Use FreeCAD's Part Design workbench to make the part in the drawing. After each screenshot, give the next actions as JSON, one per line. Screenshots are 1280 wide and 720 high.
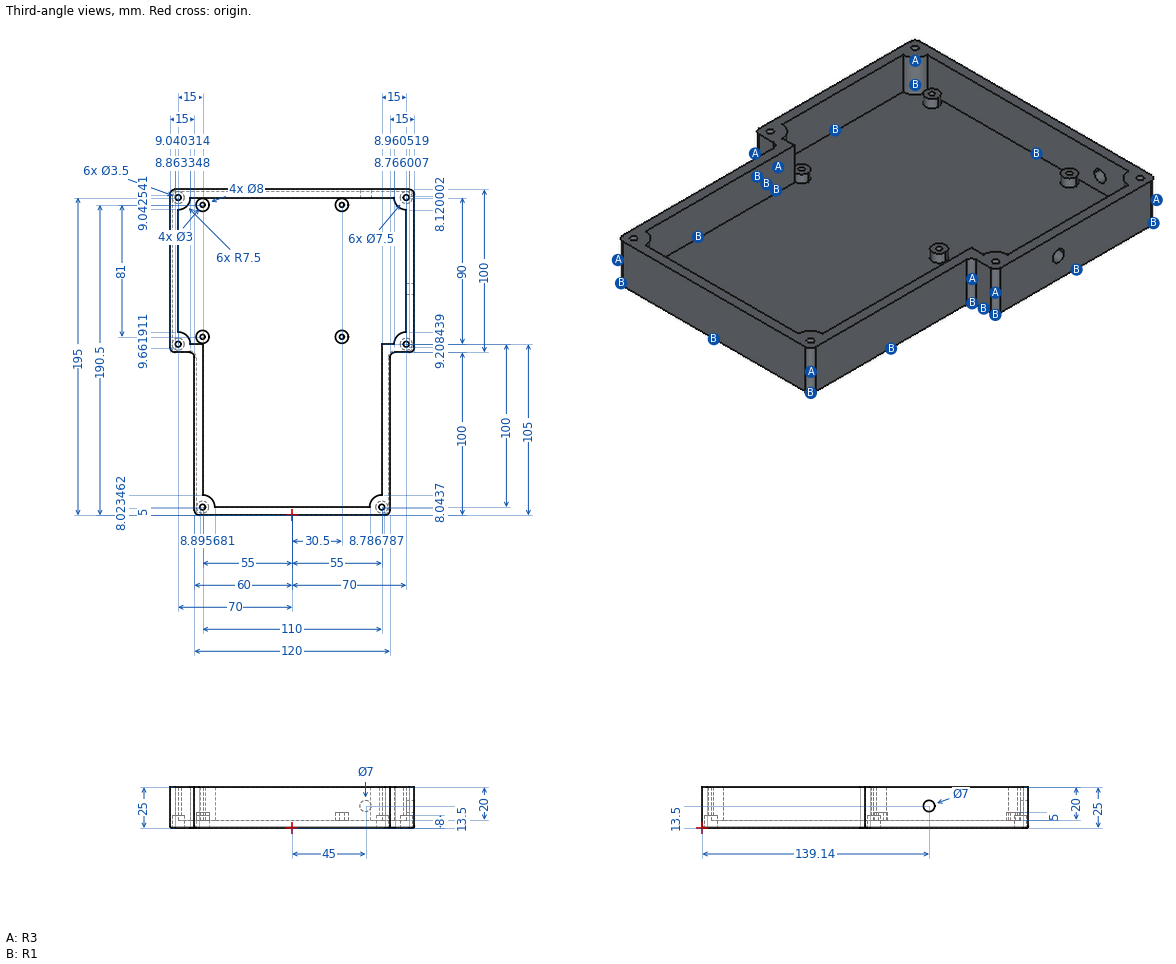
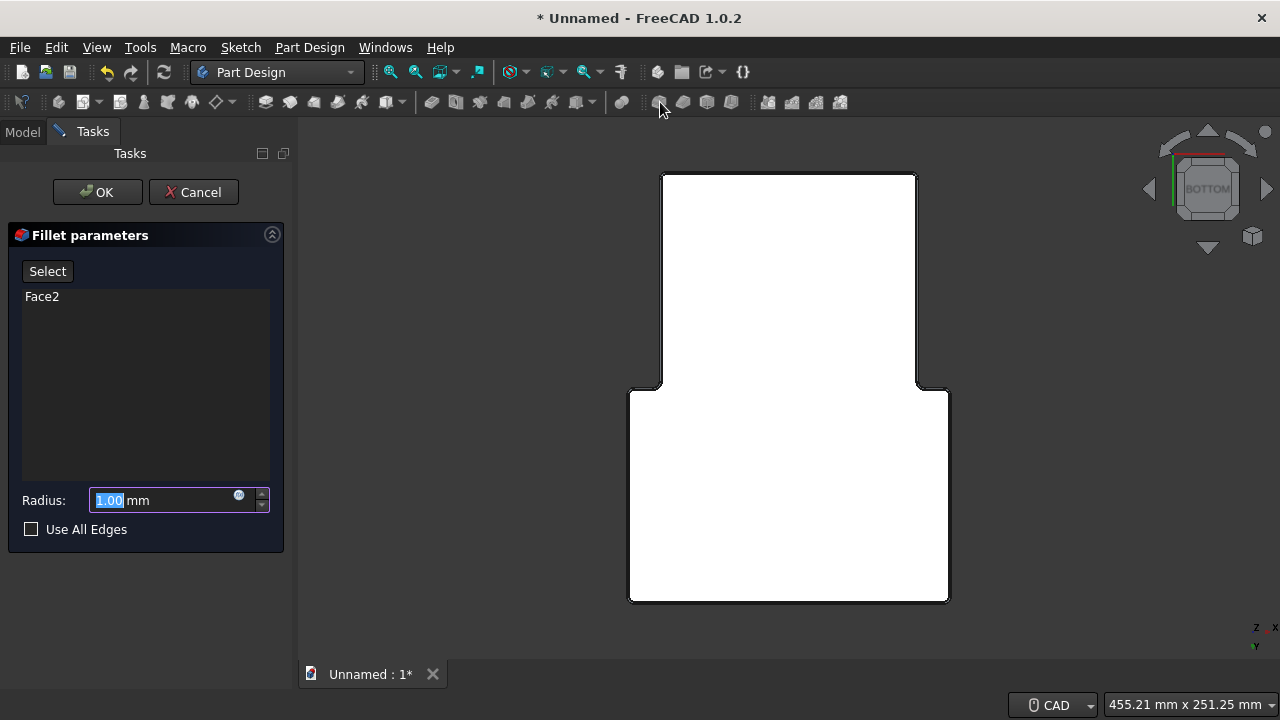
{"action": "type", "text": "1"}
{"action": "key", "text": "Tab"}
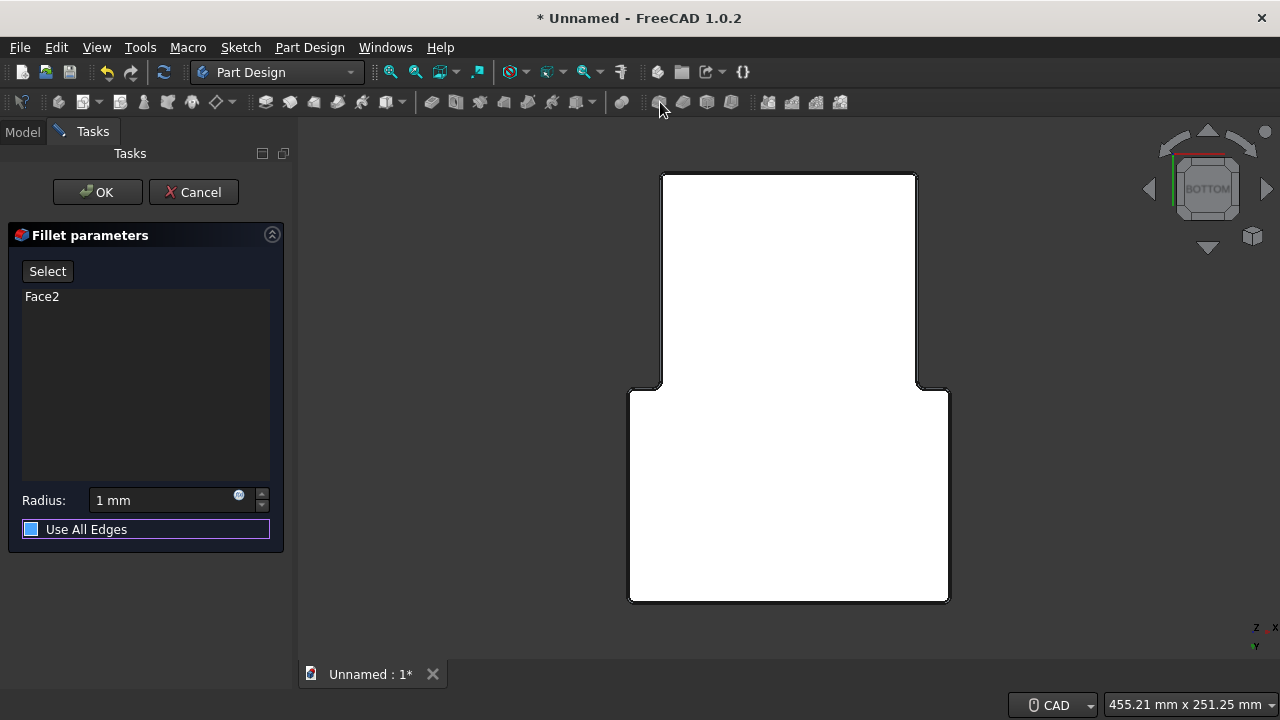
{"action": "left_click", "coordinate": [98, 192]}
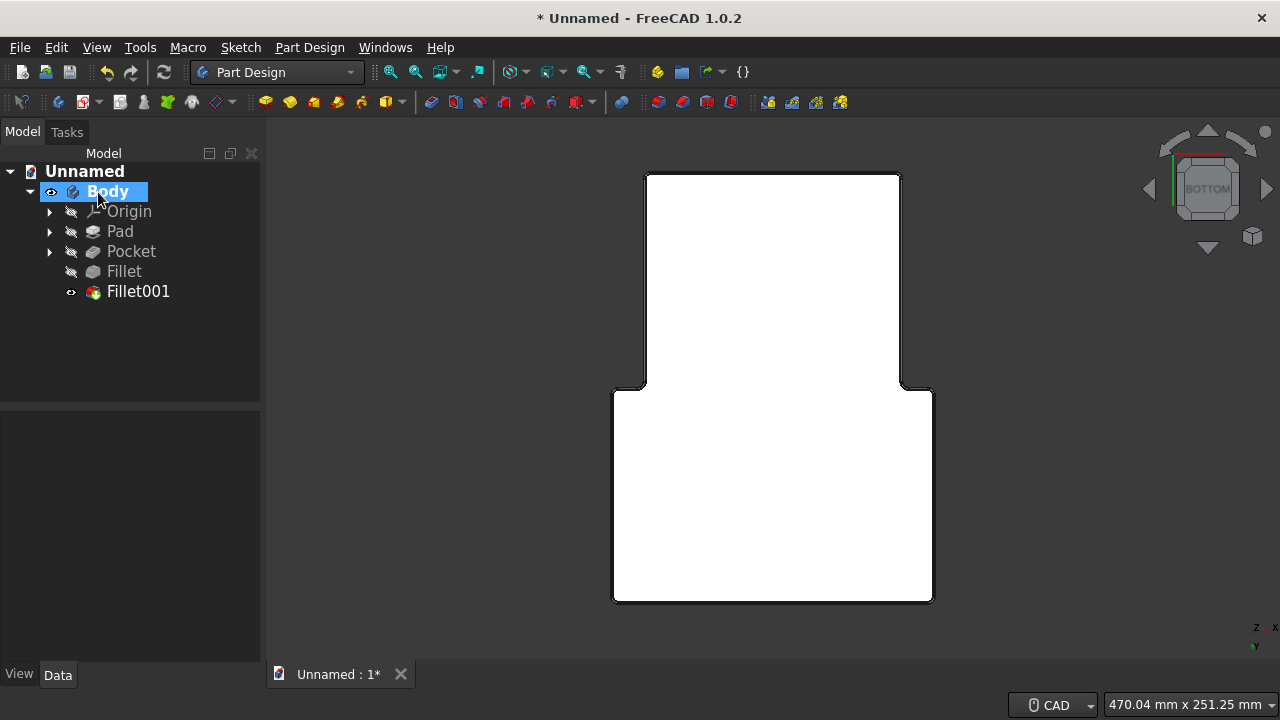
{"action": "key", "text": "0"}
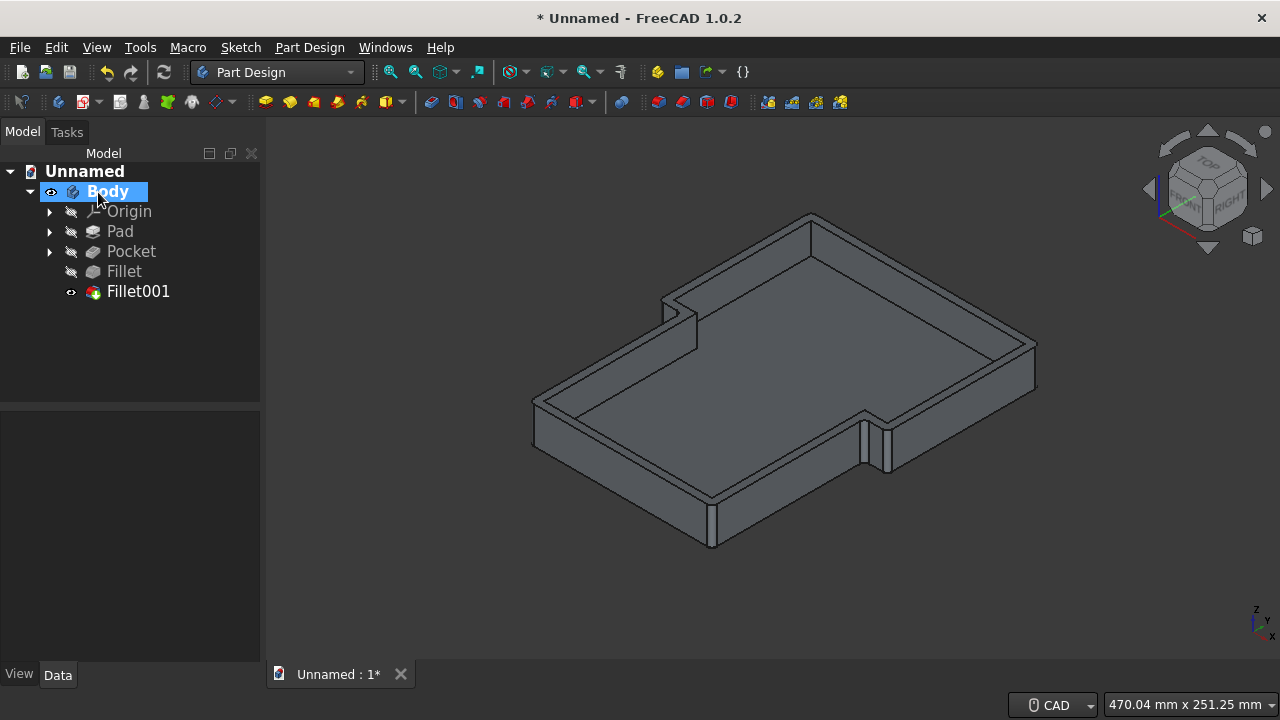
{"action": "left_click", "coordinate": [814, 376]}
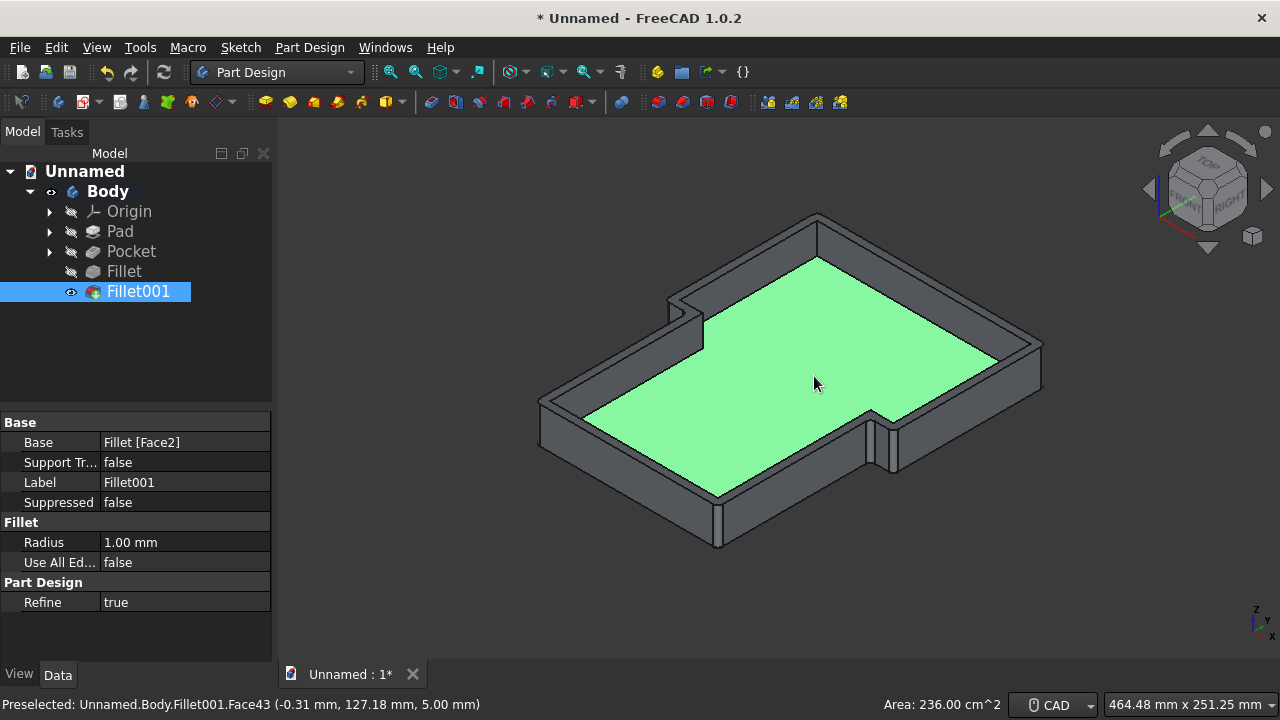
{"action": "left_click", "coordinate": [84, 102]}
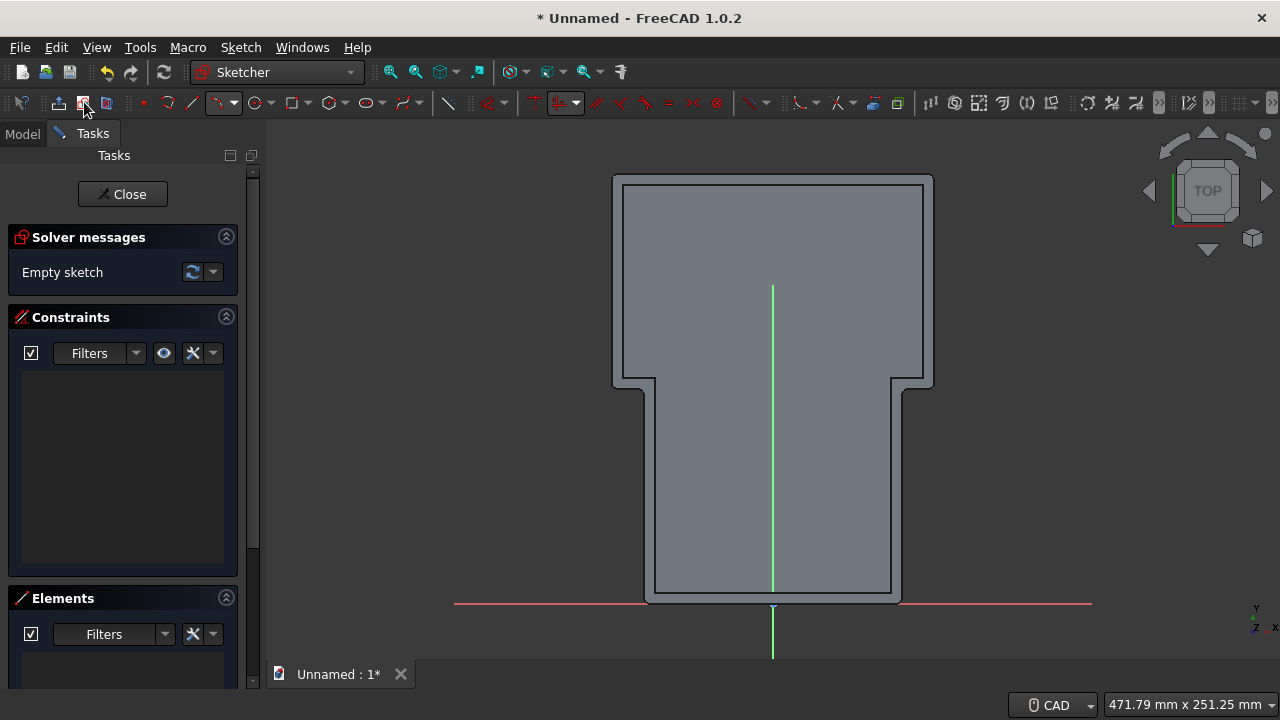
{"action": "key", "text": "g c"}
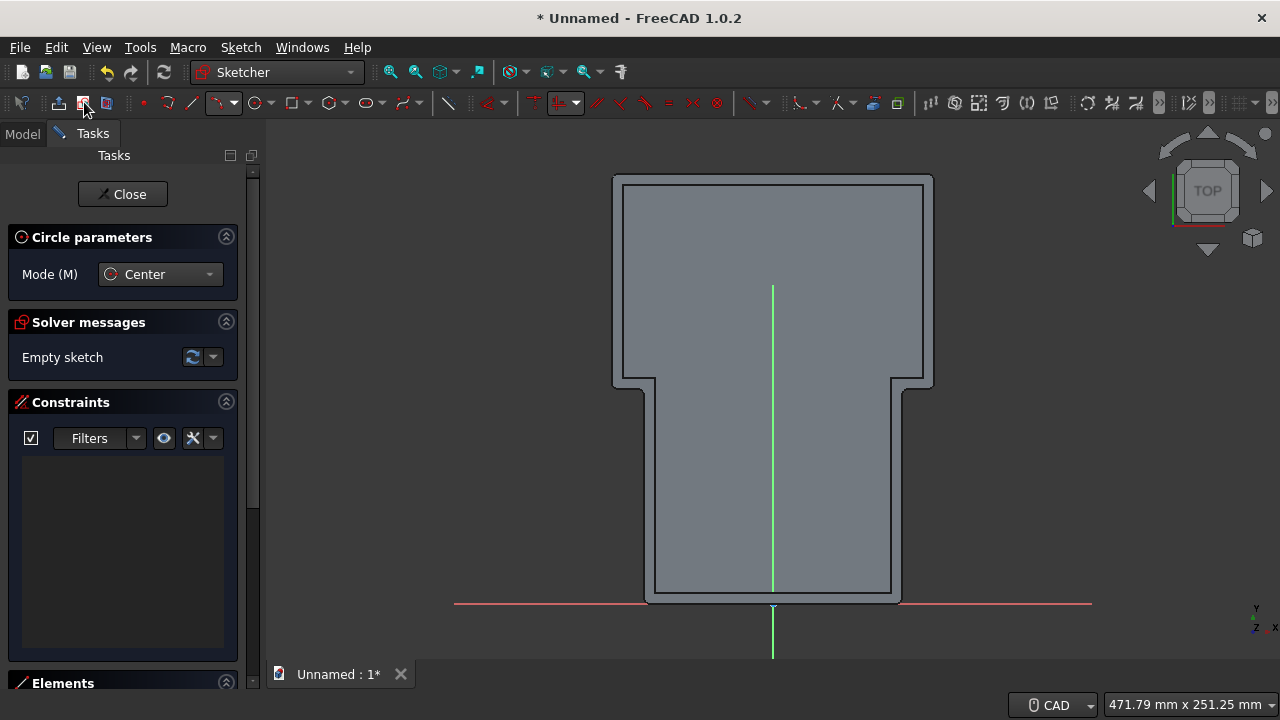
{"action": "scroll", "coordinate": [655, 194], "scroll_direction": "up", "scroll_amount": 5}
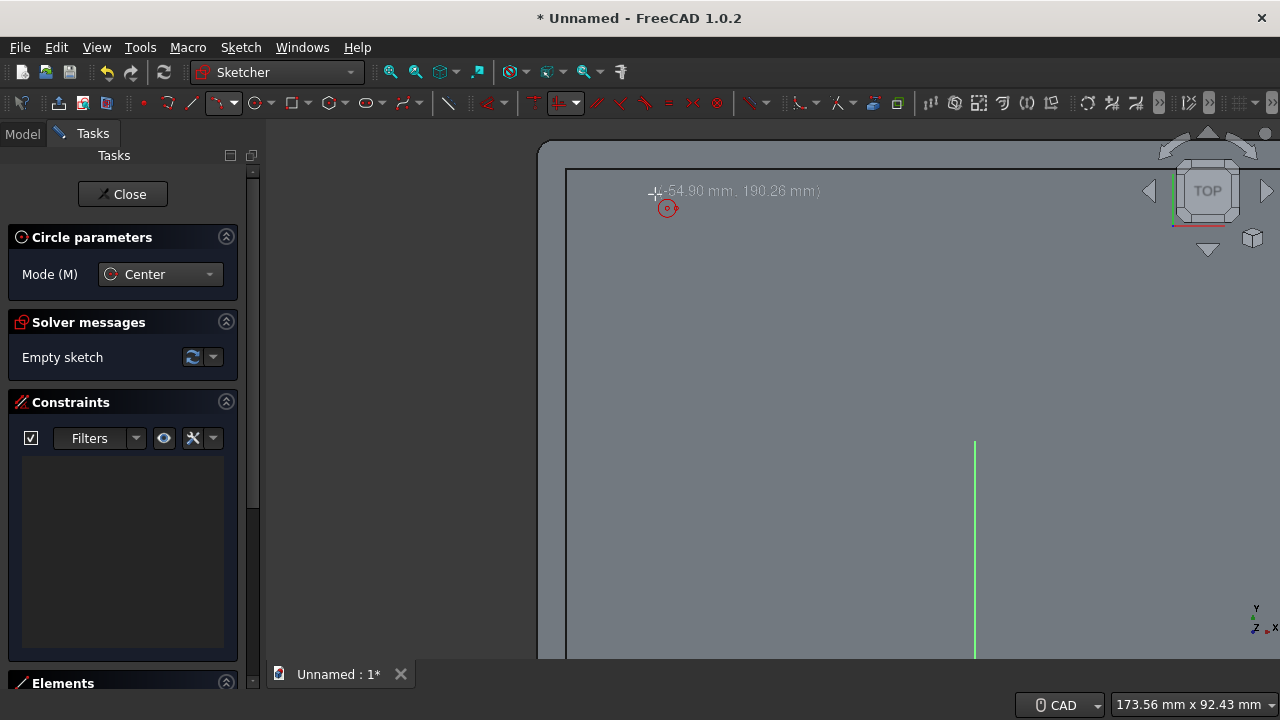
{"action": "left_click", "coordinate": [654, 195]}
{"action": "mouse_move", "coordinate": [670, 179]}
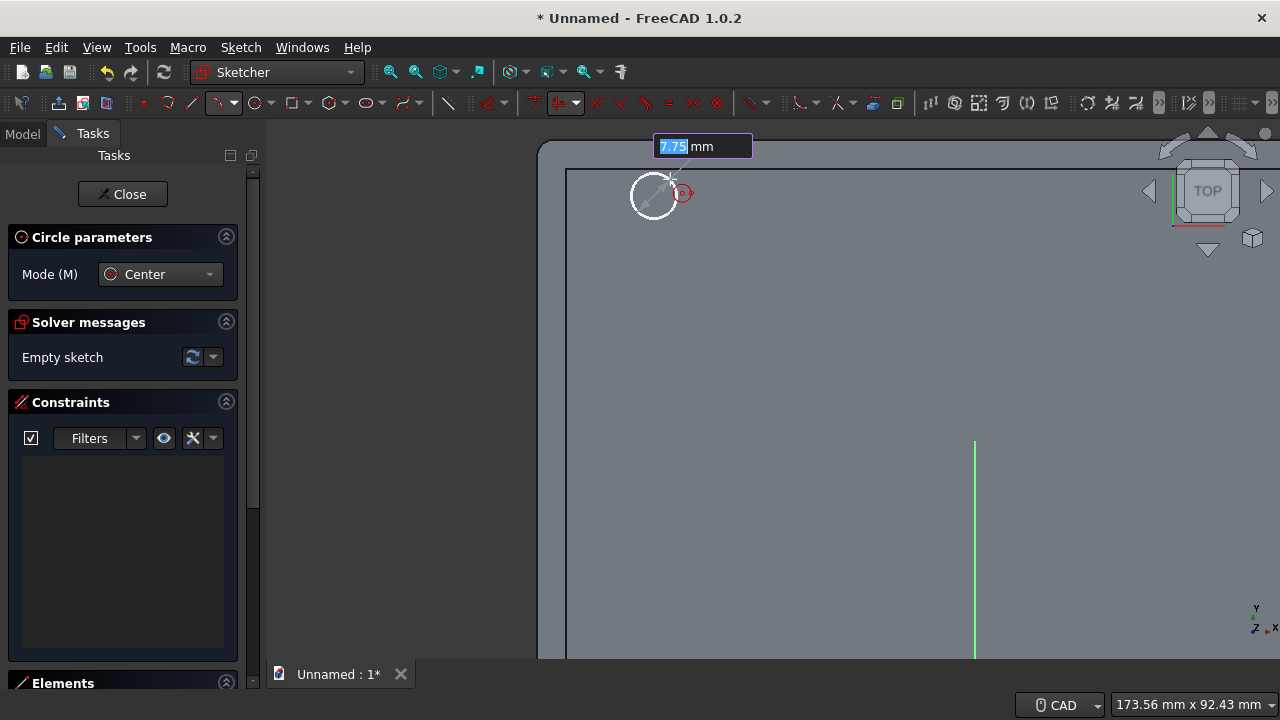
{"action": "type", "text": "8"}
{"action": "key", "text": "Return"}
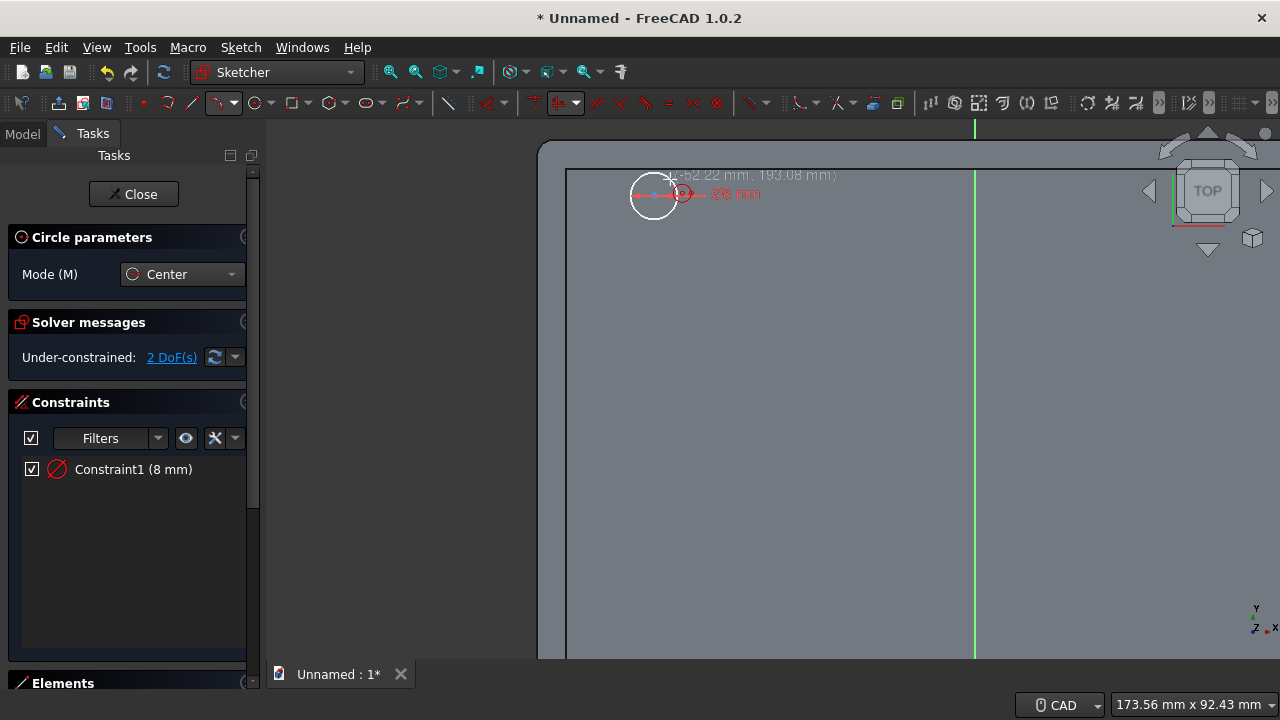
{"action": "scroll", "coordinate": [619, 238], "scroll_direction": "down", "scroll_amount": 6}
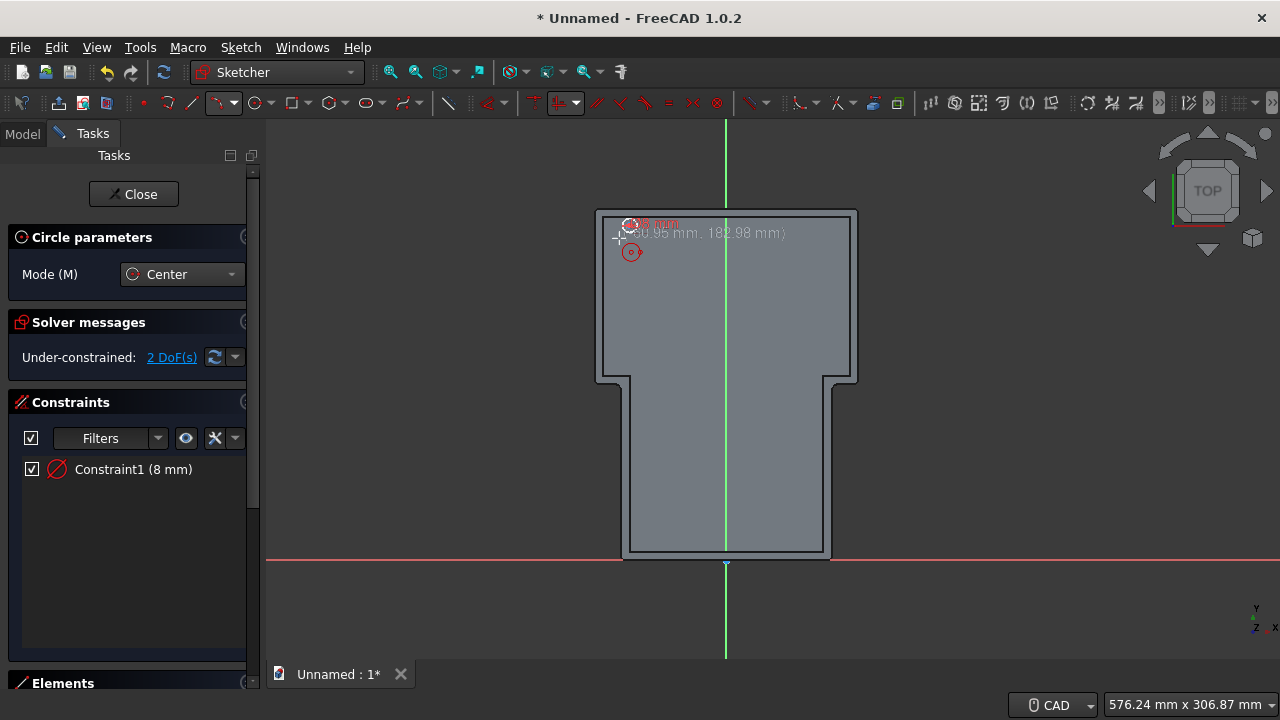
{"action": "scroll", "coordinate": [780, 225], "scroll_direction": "up", "scroll_amount": 6}